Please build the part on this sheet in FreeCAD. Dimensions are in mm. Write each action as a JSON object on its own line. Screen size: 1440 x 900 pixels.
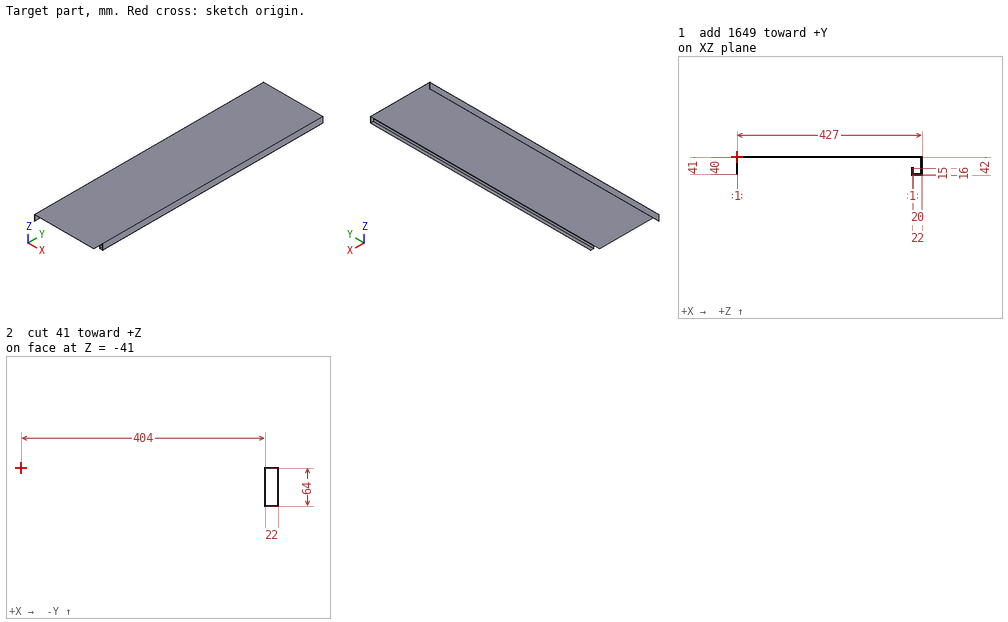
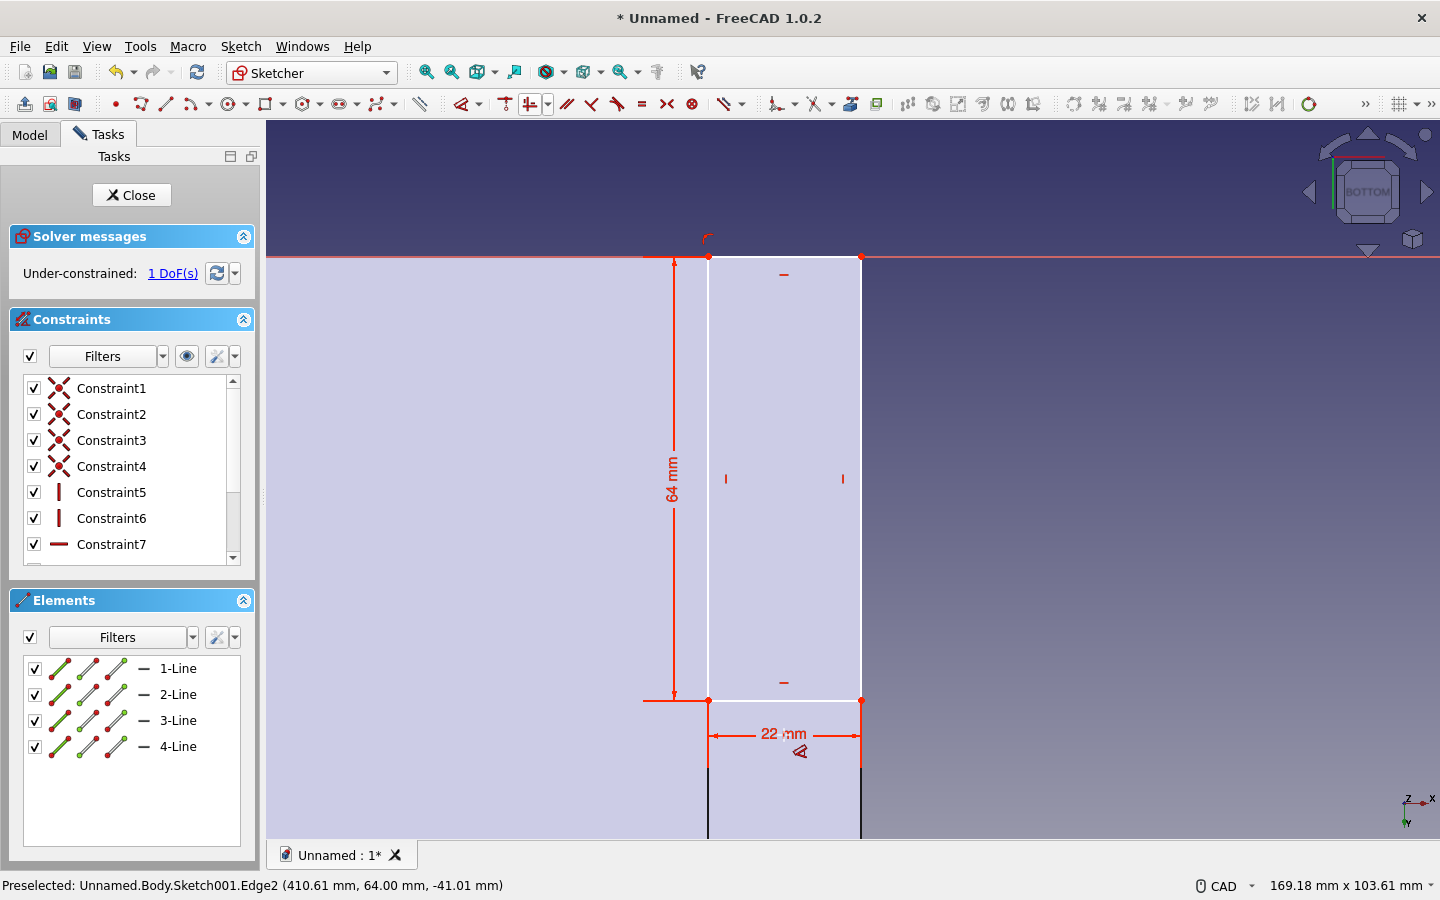
{"action": "left_click", "coordinate": [708, 257]}
{"action": "left_click", "coordinate": [501, 223]}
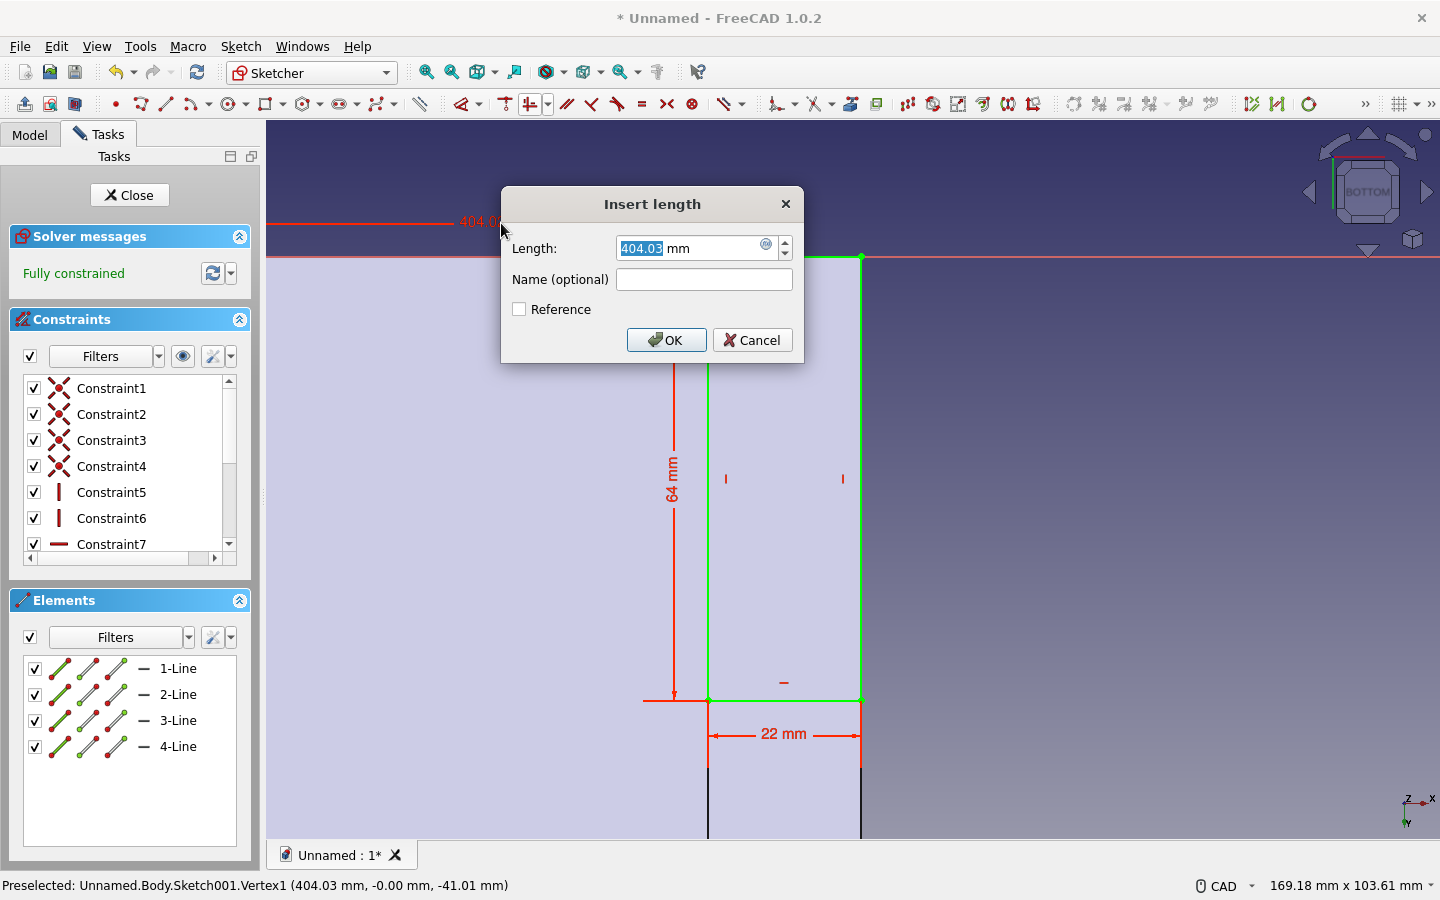
{"action": "type", "text": "404"}
{"action": "key", "text": "Return"}
{"action": "key", "text": "Escape"}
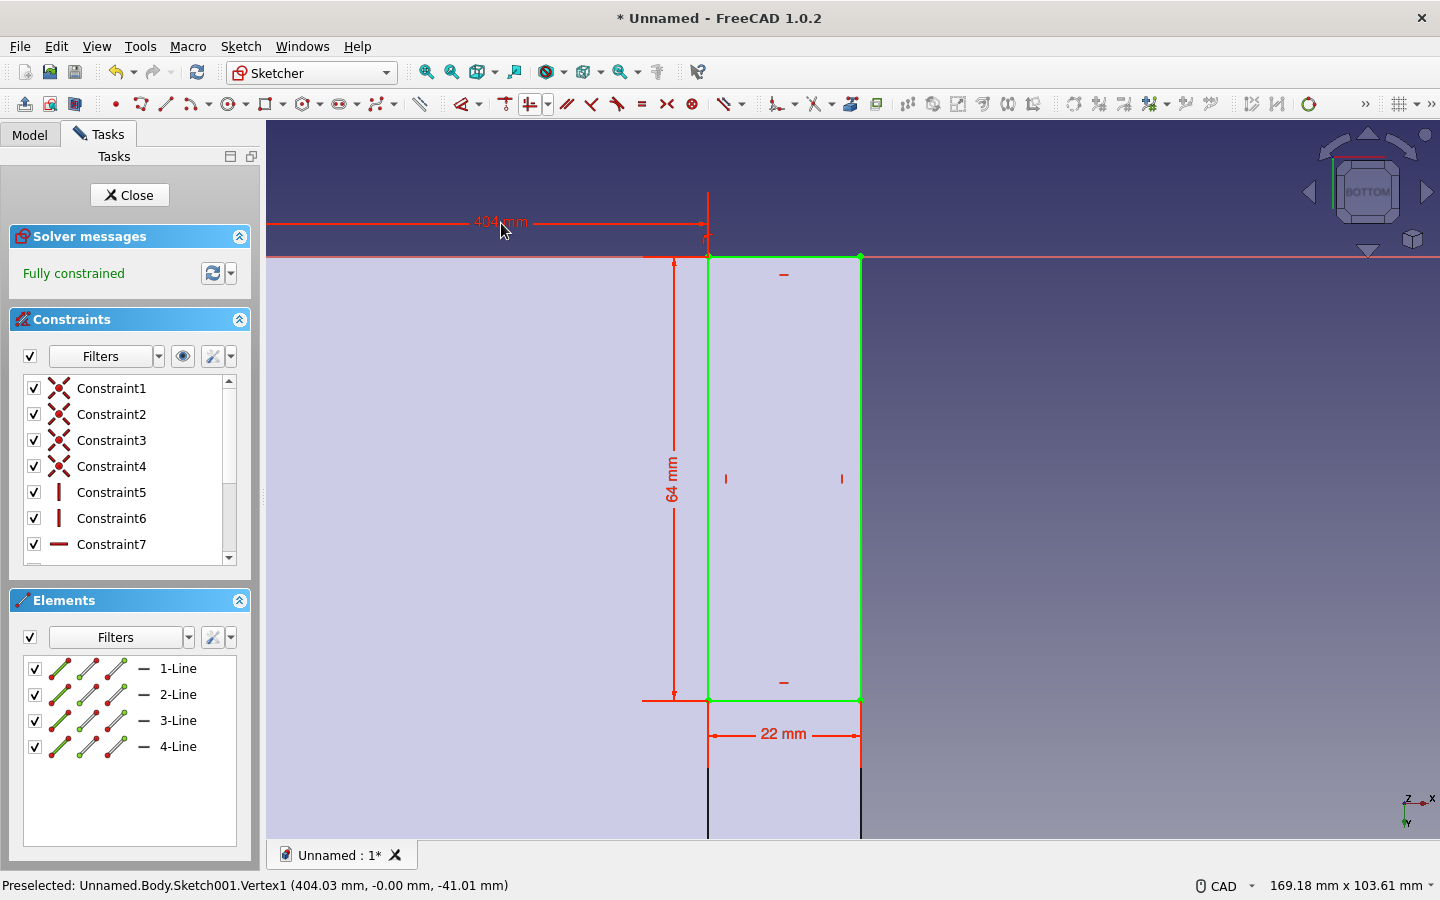
{"action": "left_click", "coordinate": [130, 195]}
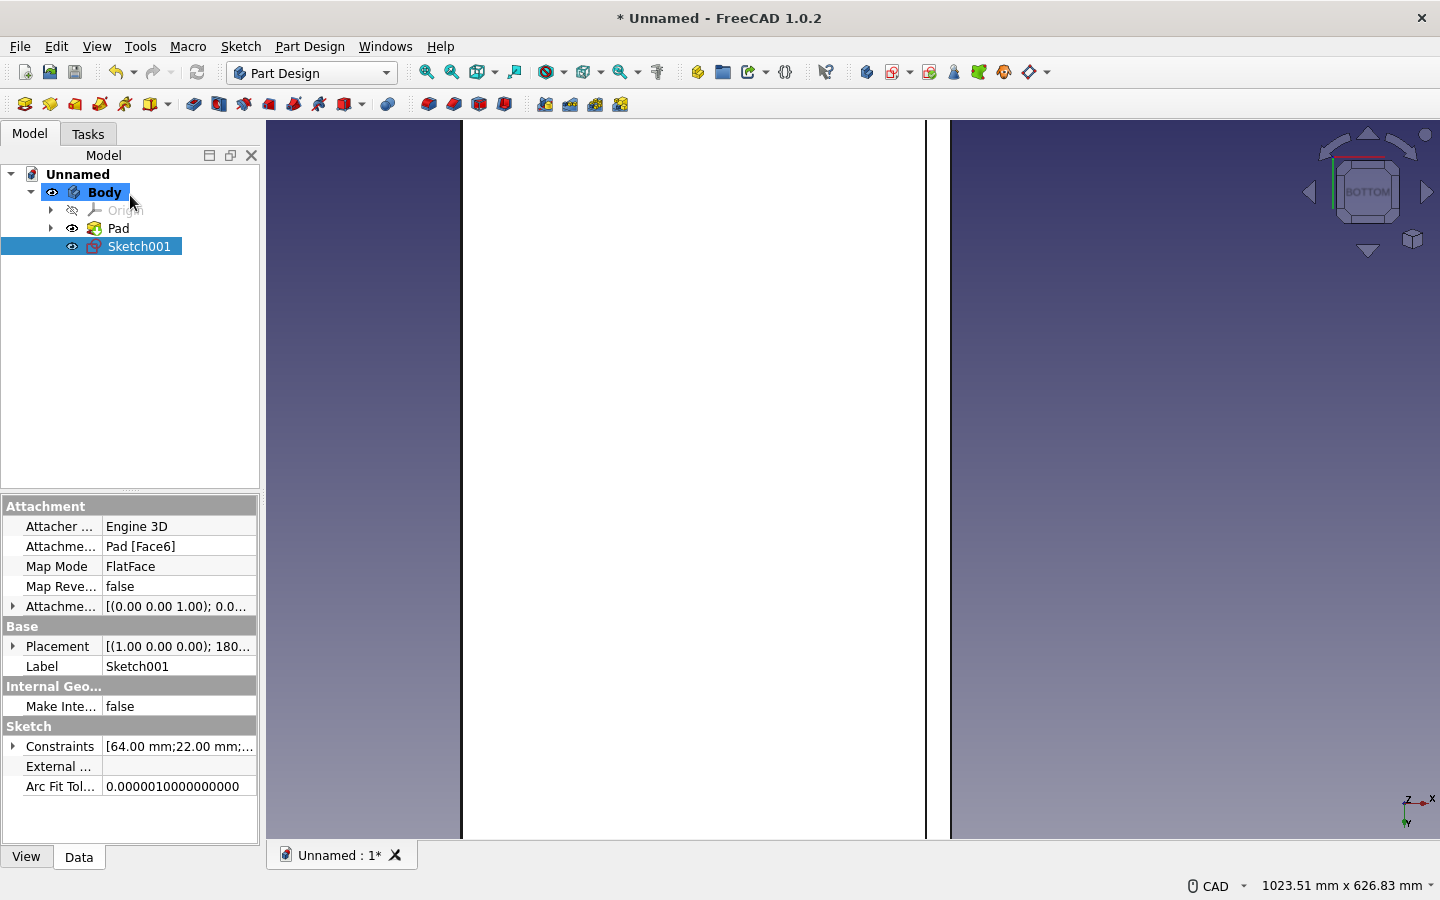
{"action": "left_click", "coordinate": [194, 104]}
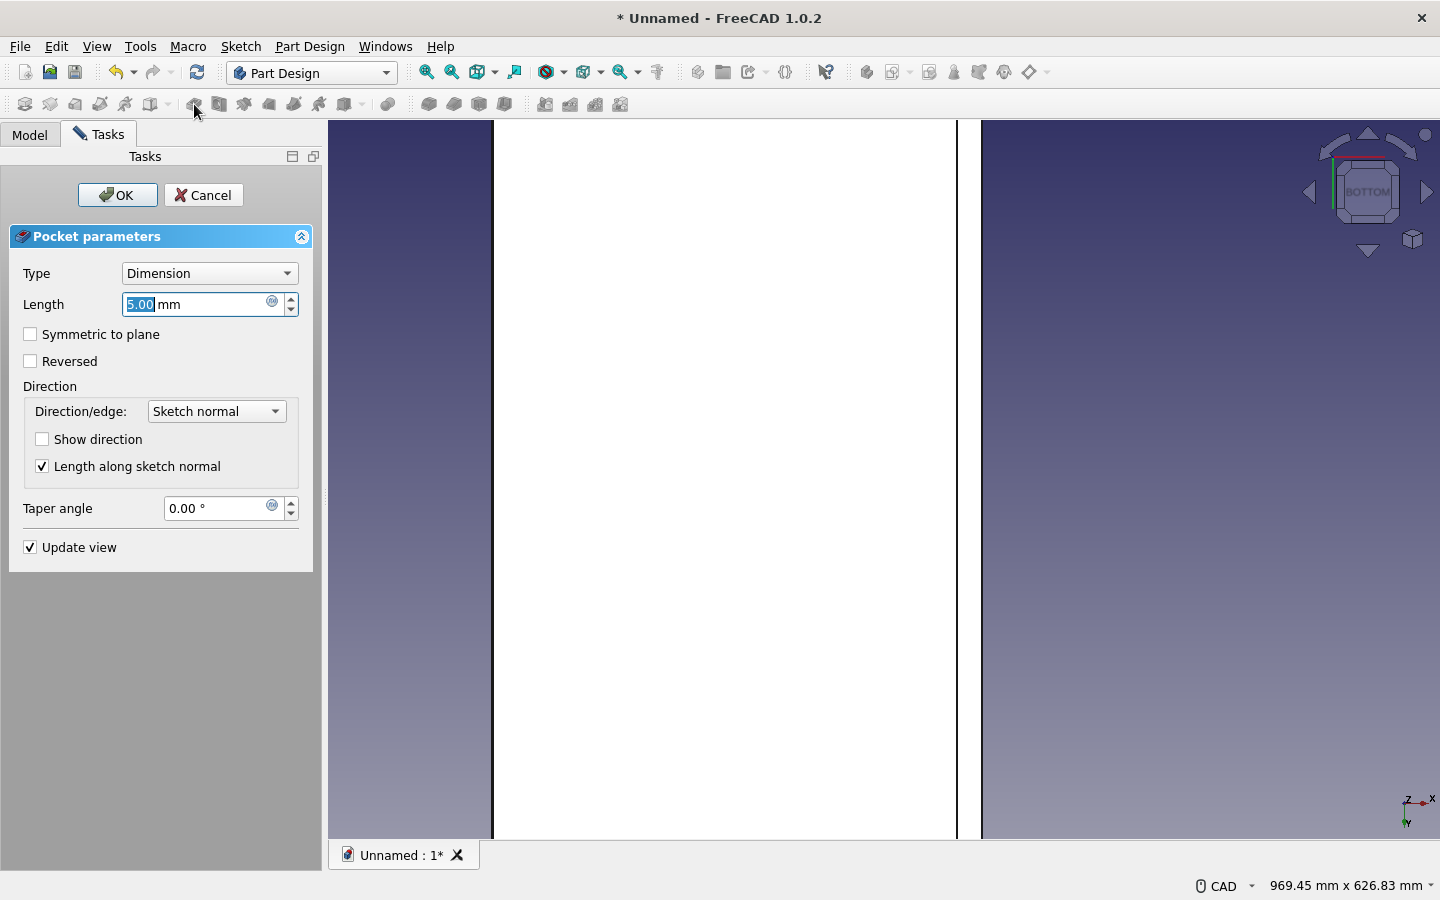
{"action": "type", "text": "41"}
{"action": "key", "text": "Tab"}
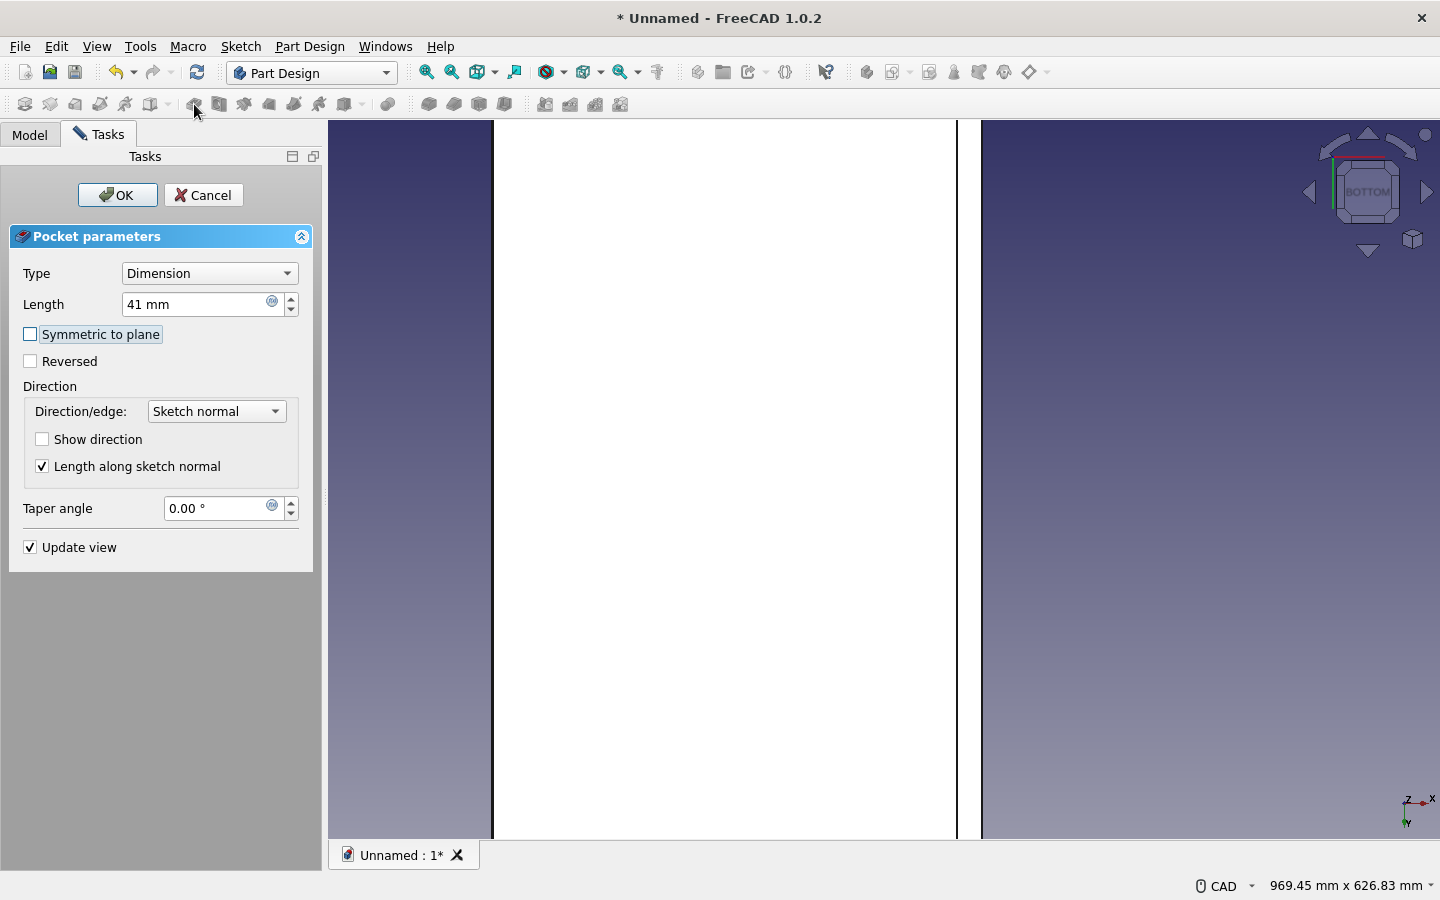
{"action": "left_click", "coordinate": [118, 195]}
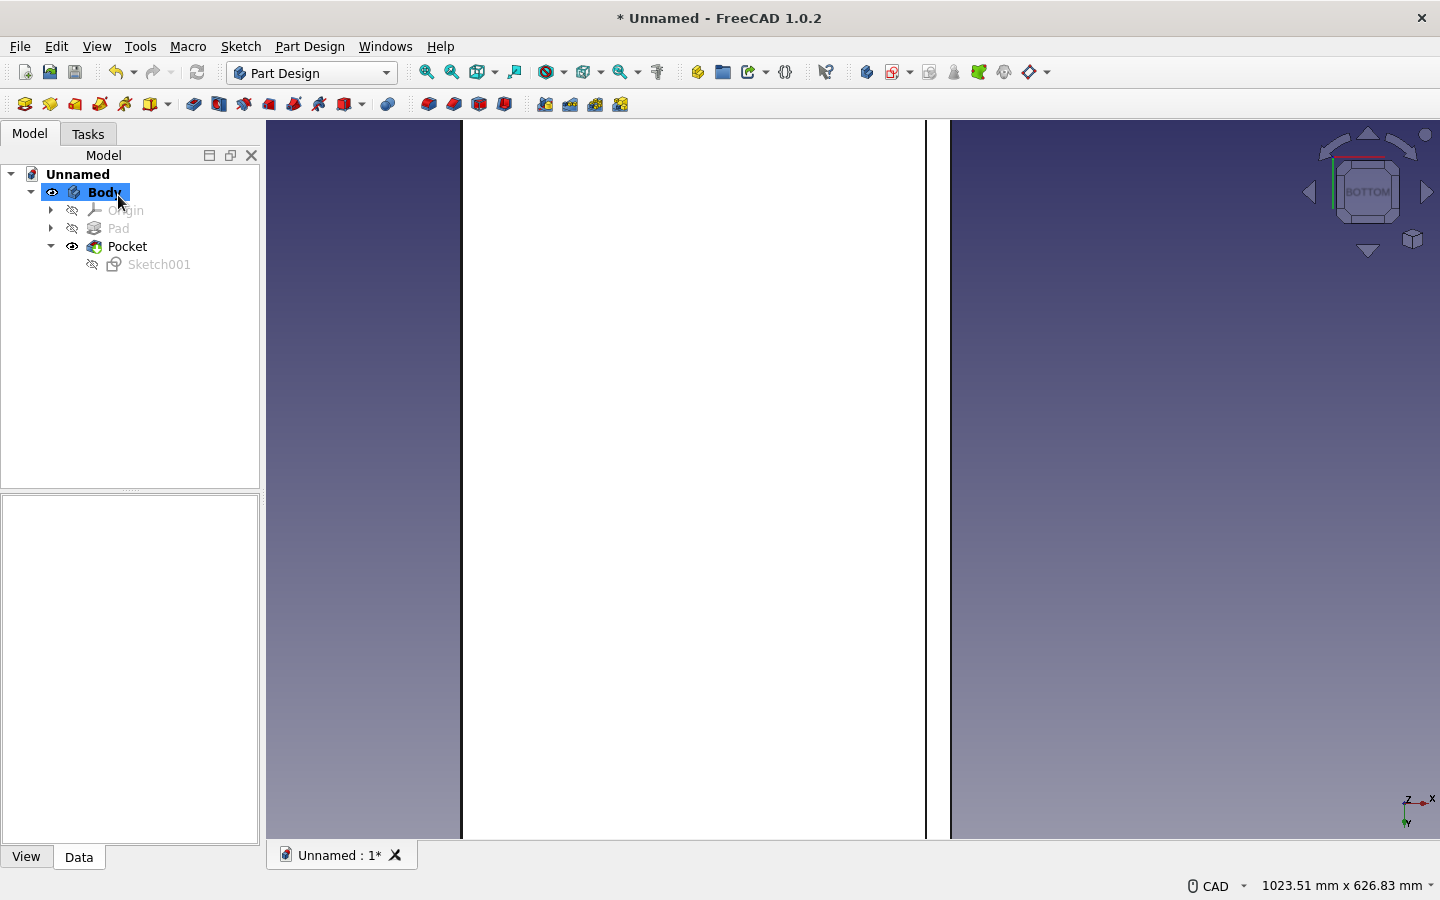
{"action": "key", "text": "0"}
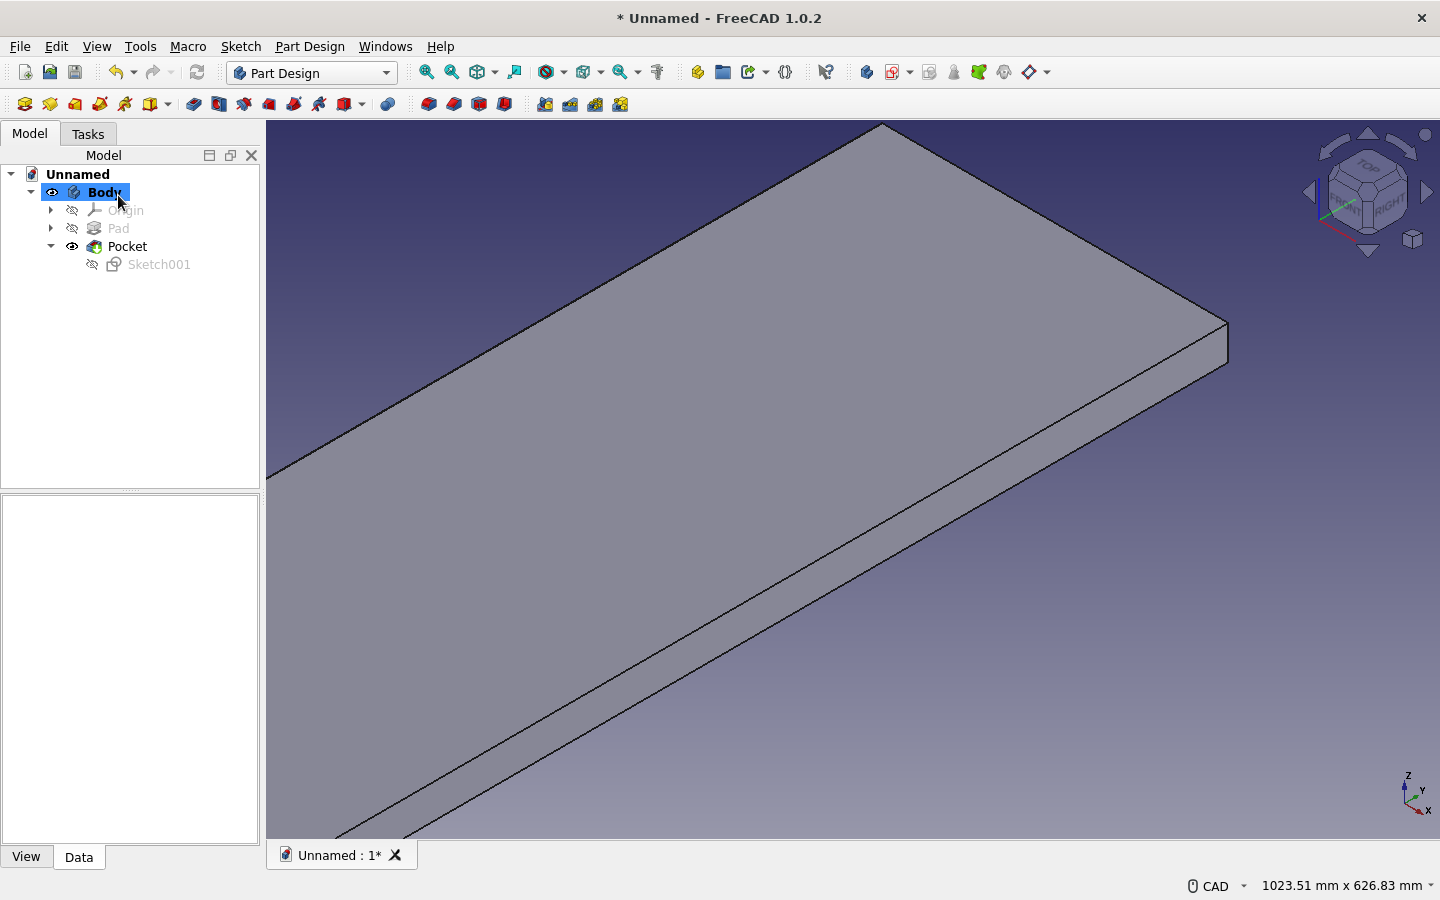
{"action": "left_click", "coordinate": [427, 72]}